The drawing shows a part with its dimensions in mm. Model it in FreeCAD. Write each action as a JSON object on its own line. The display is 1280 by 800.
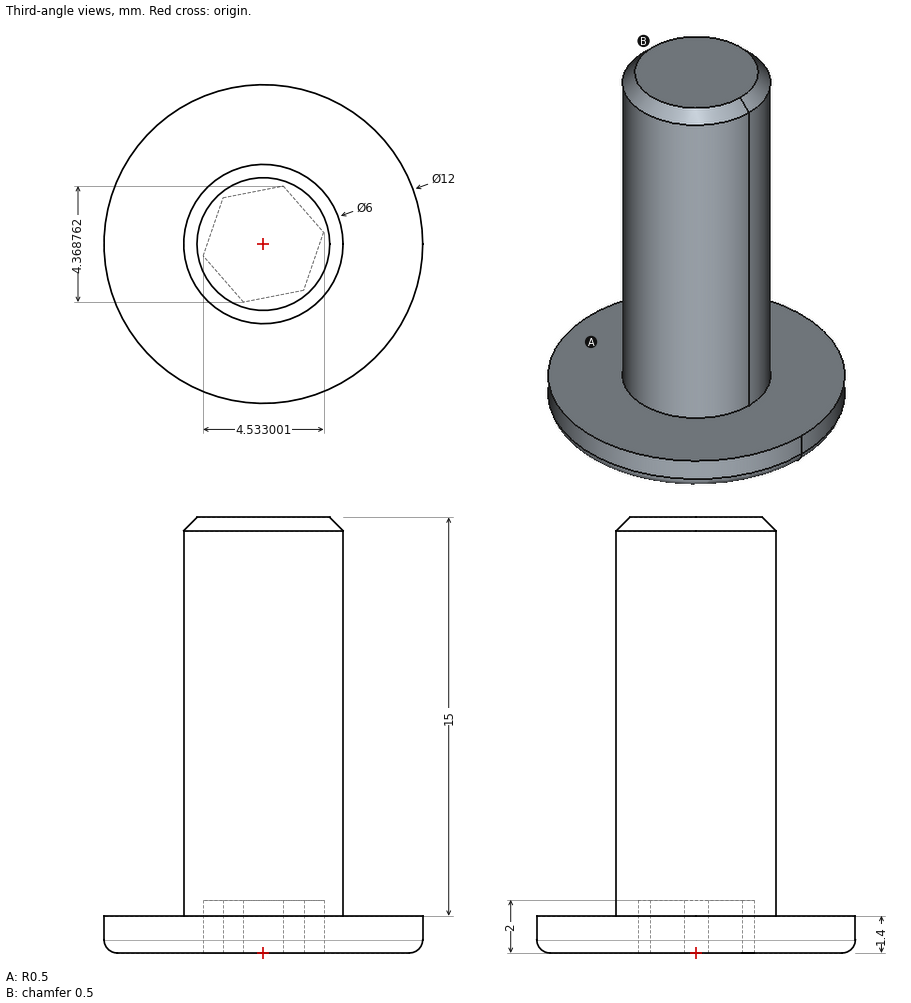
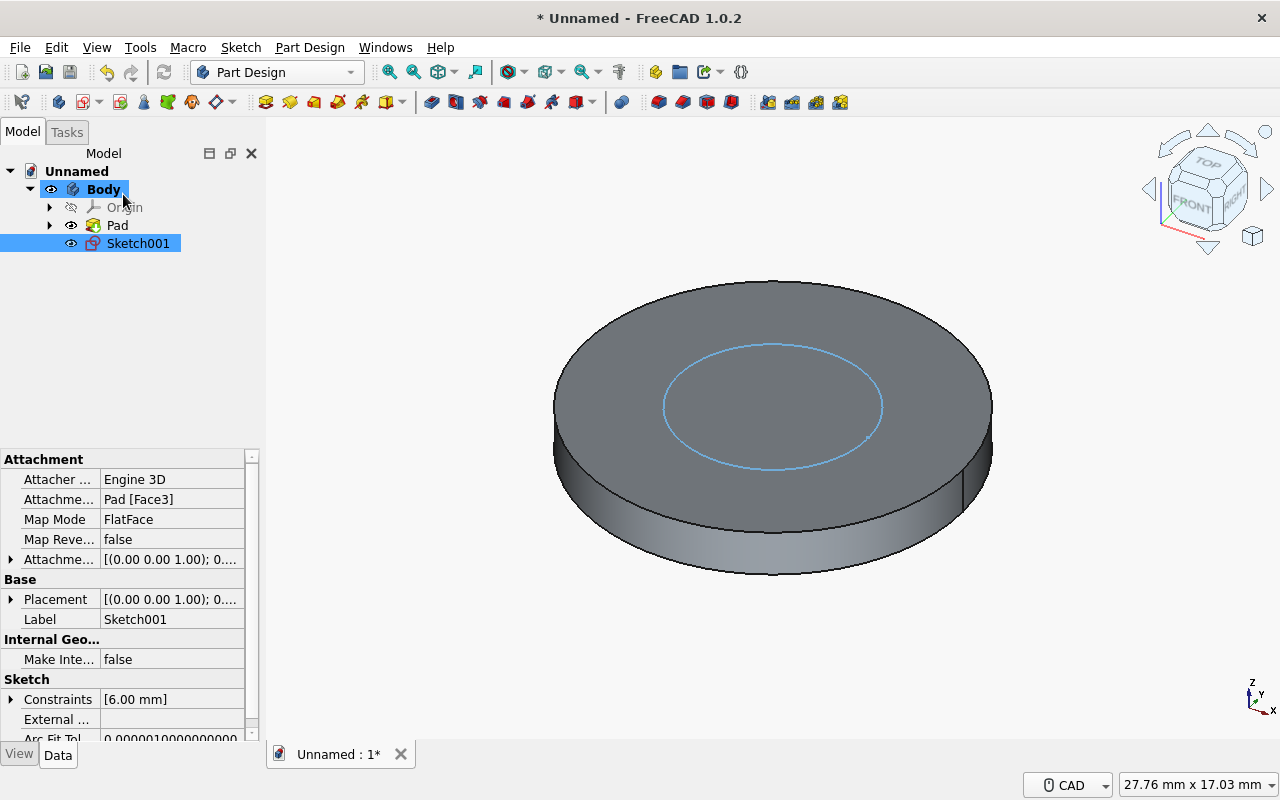
{"action": "left_click", "coordinate": [266, 102]}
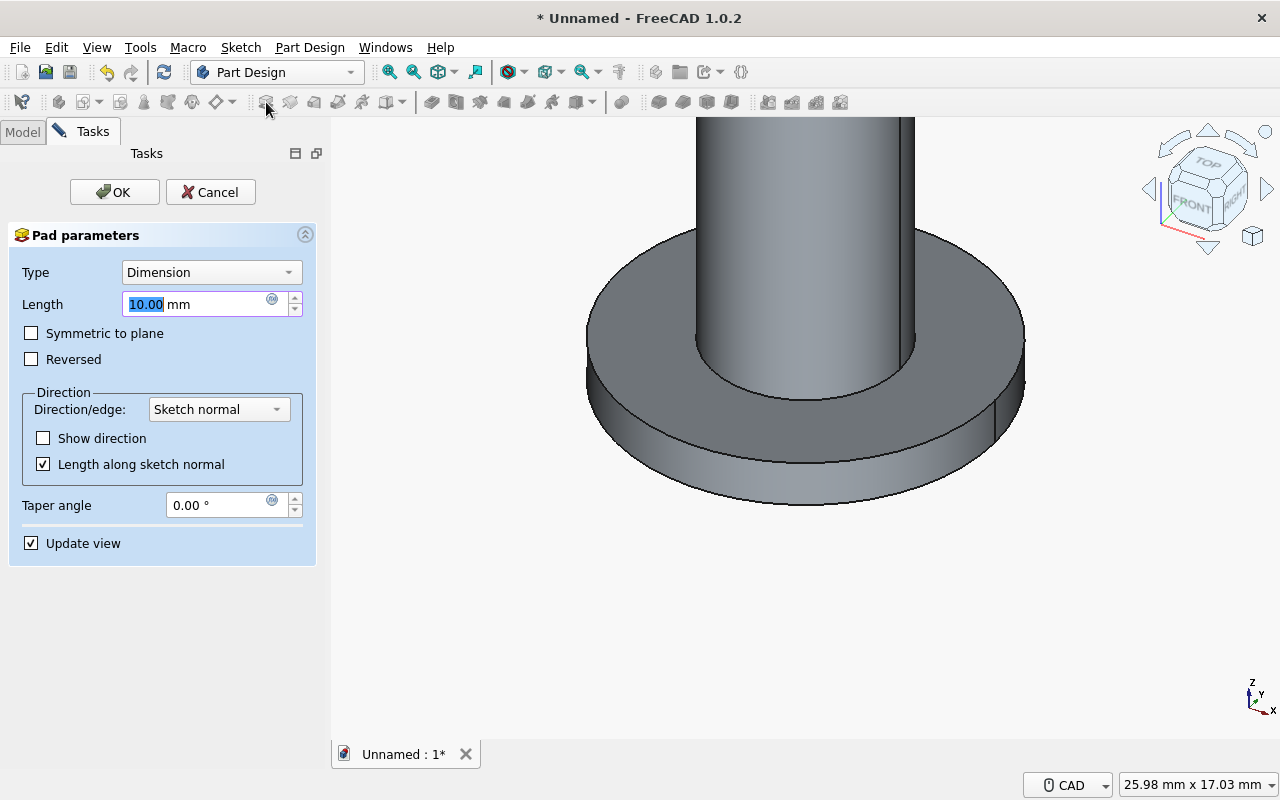
{"action": "type", "text": "15"}
{"action": "key", "text": "Tab"}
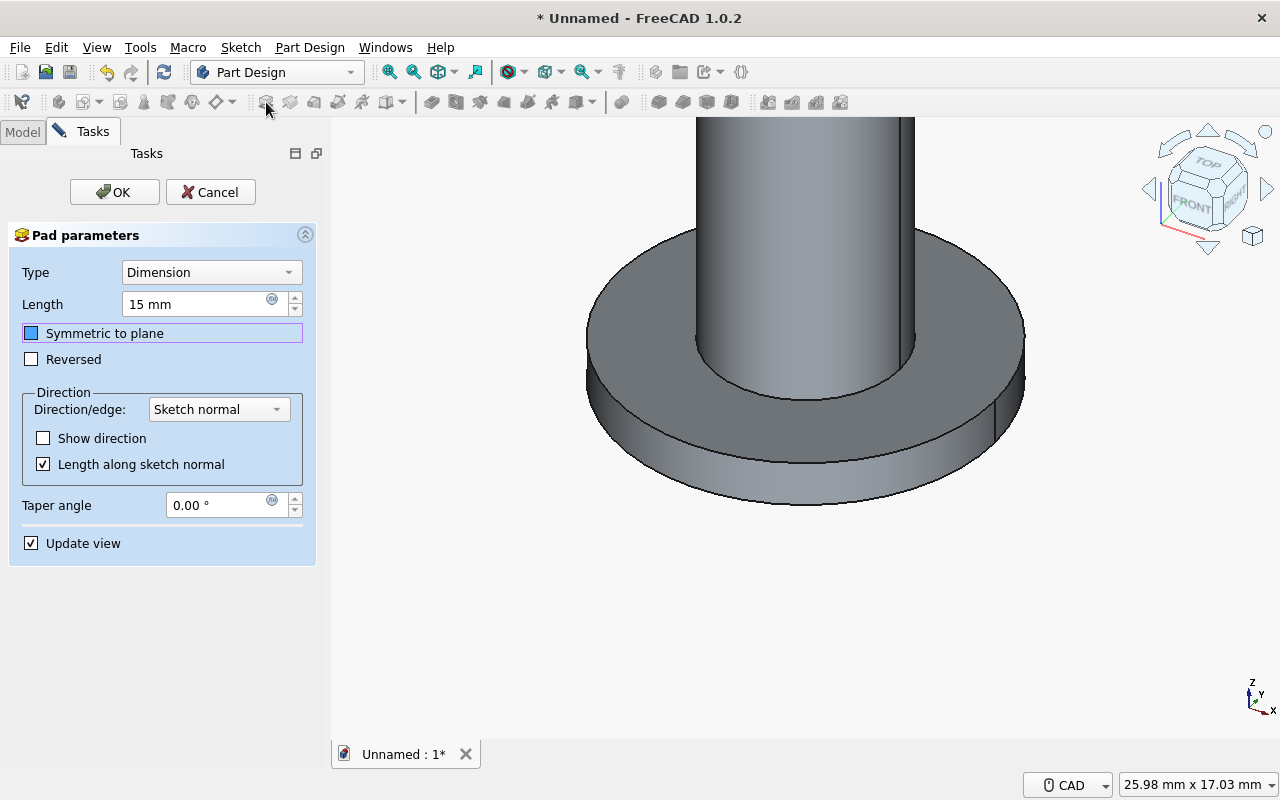
{"action": "left_click", "coordinate": [115, 192]}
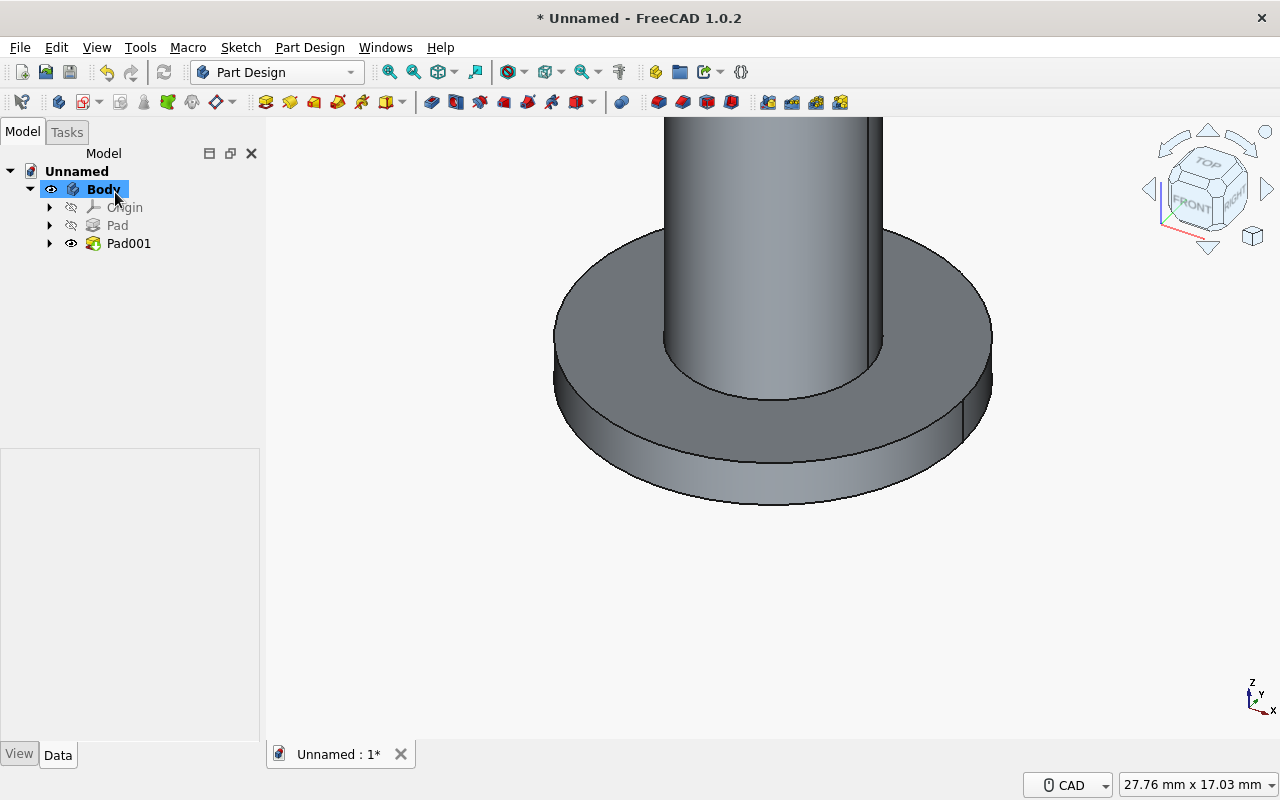
{"action": "left_click", "coordinate": [390, 72]}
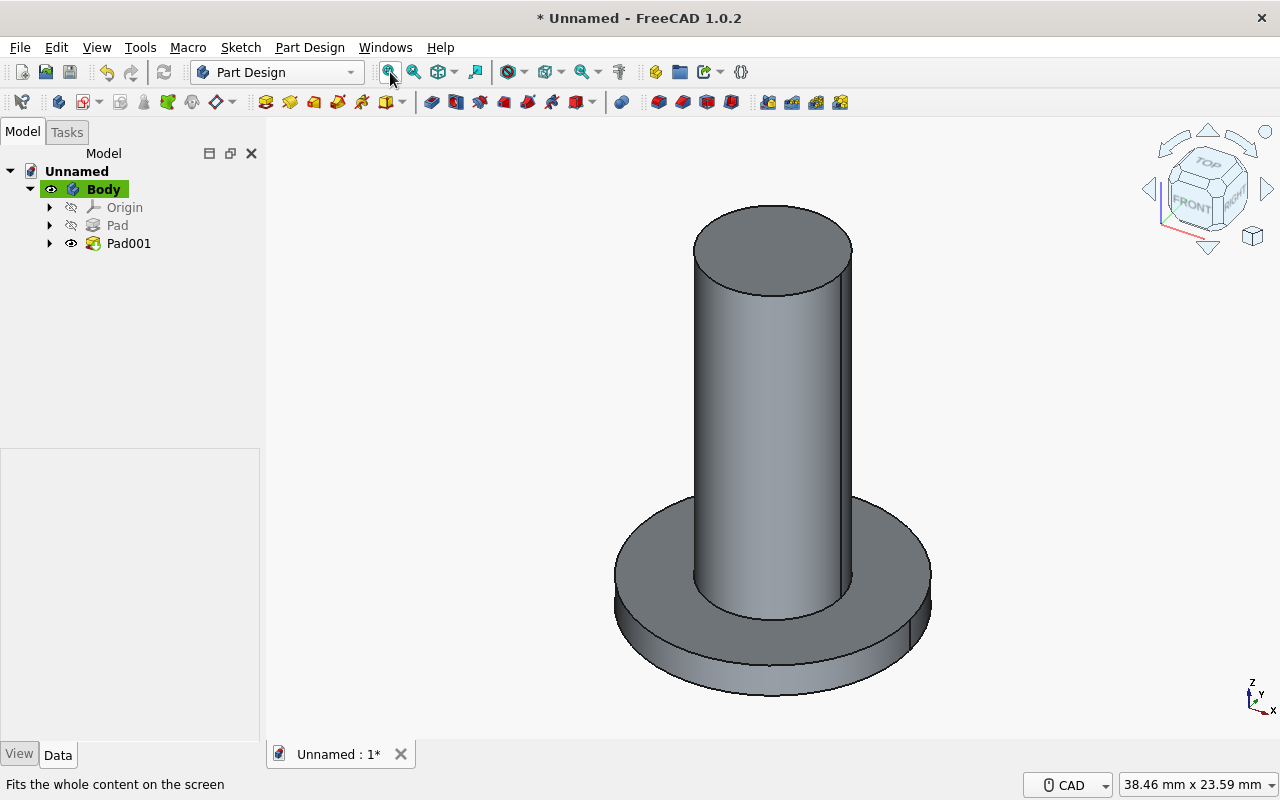
{"action": "key", "text": "0"}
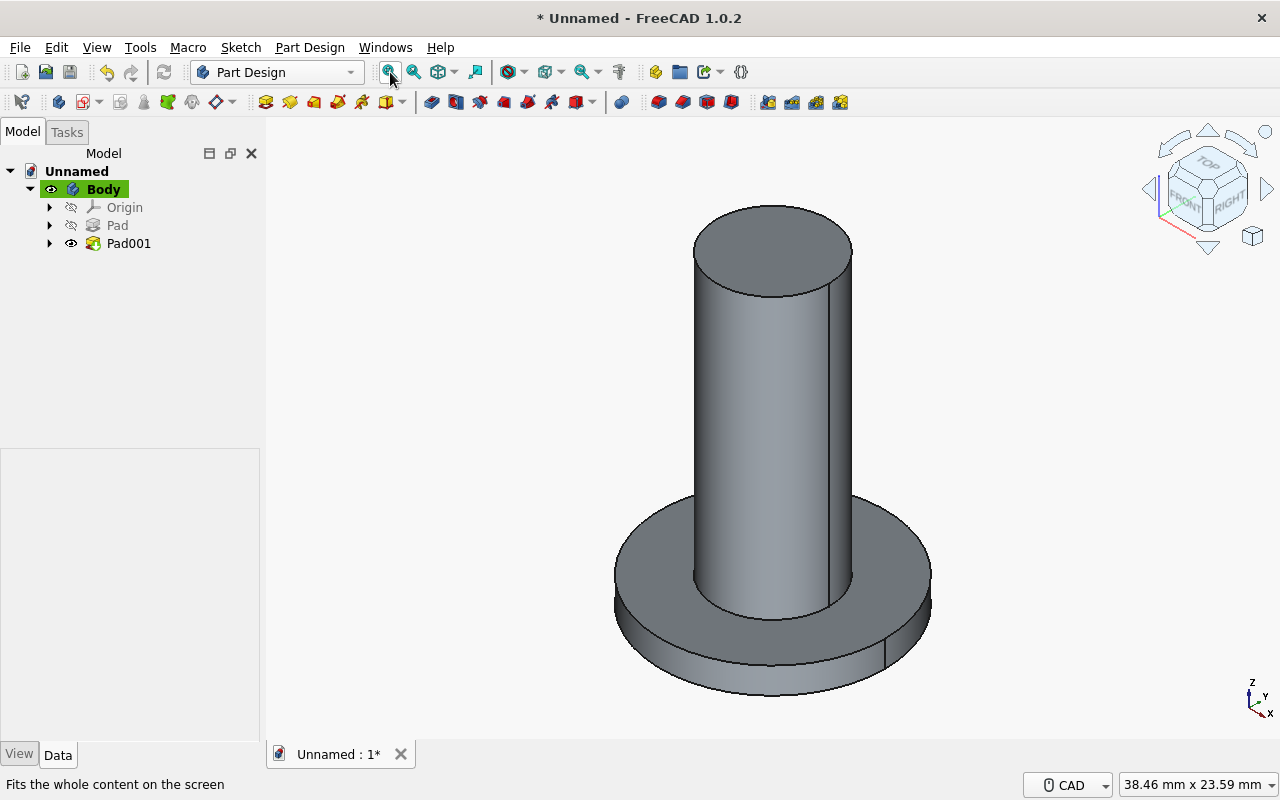
{"action": "key", "text": "2"}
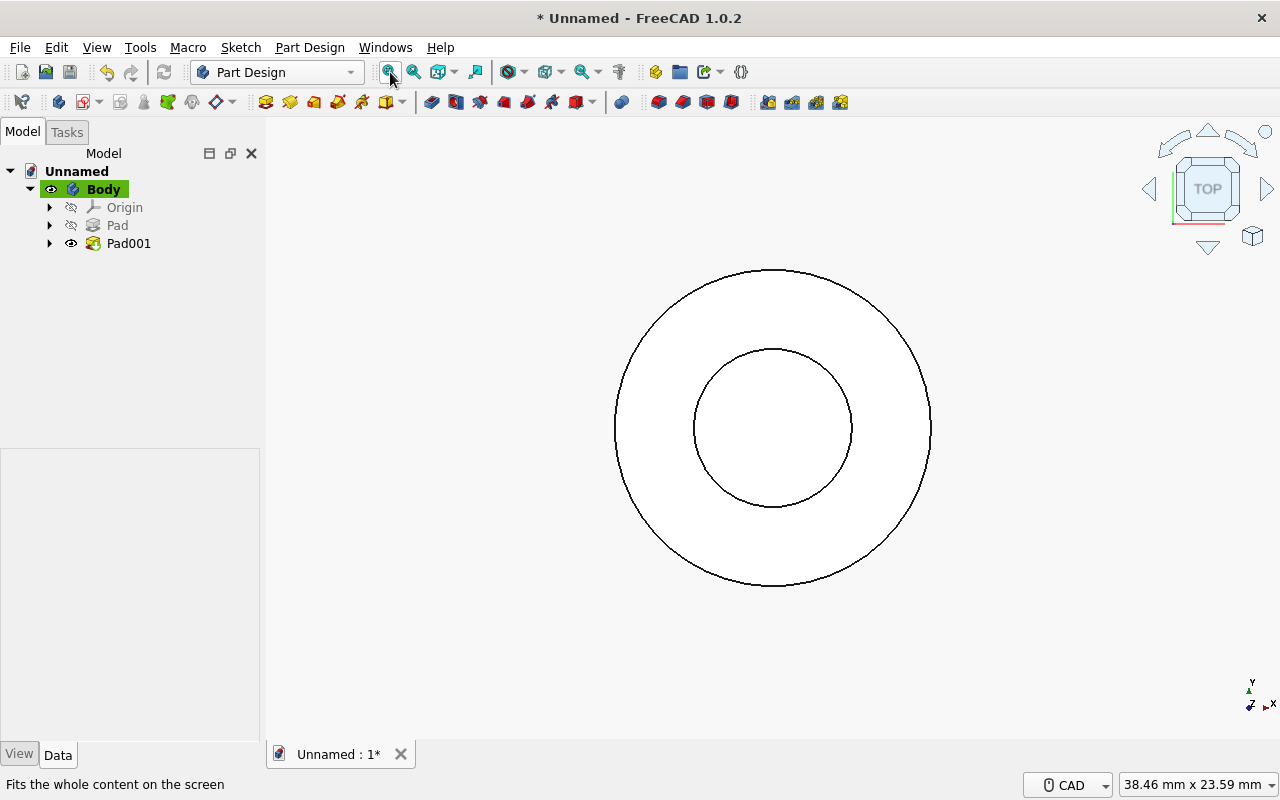
{"action": "key", "text": "1"}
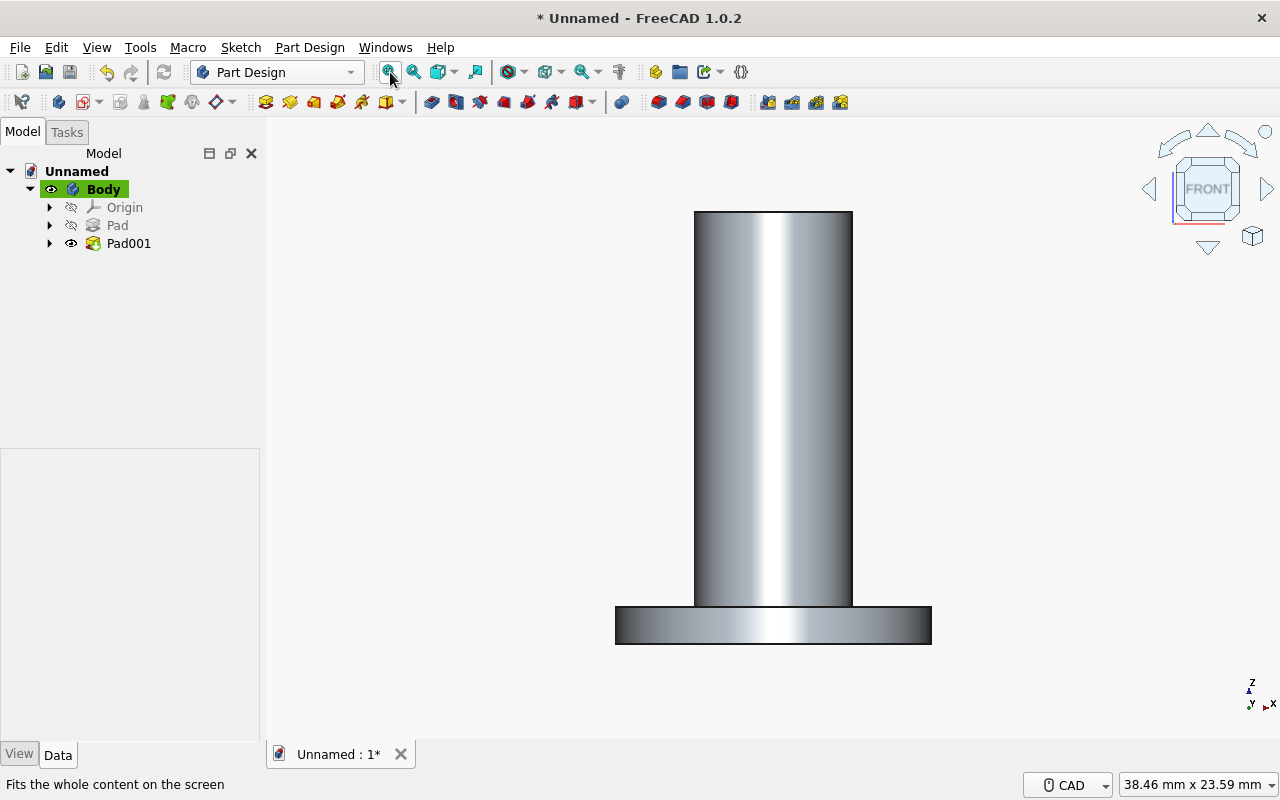
{"action": "left_click", "coordinate": [645, 643]}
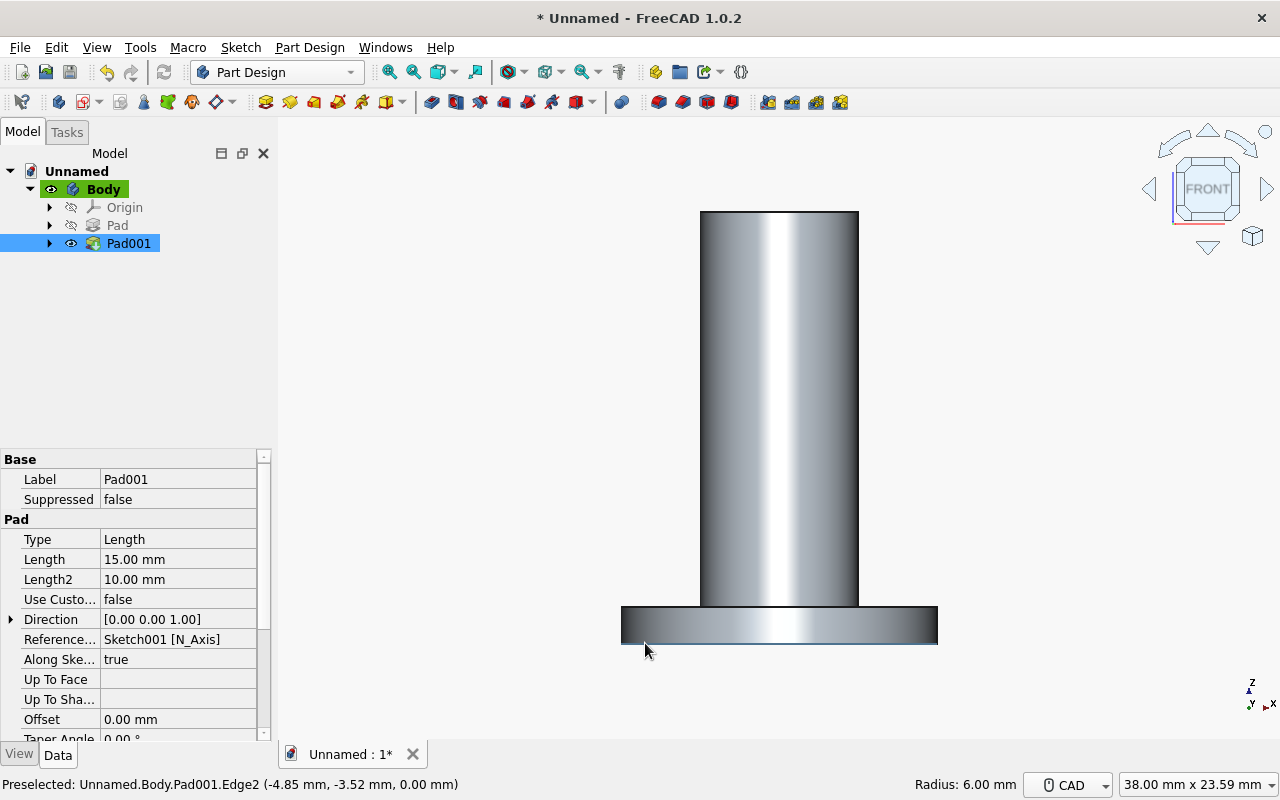
{"action": "left_click", "coordinate": [660, 102]}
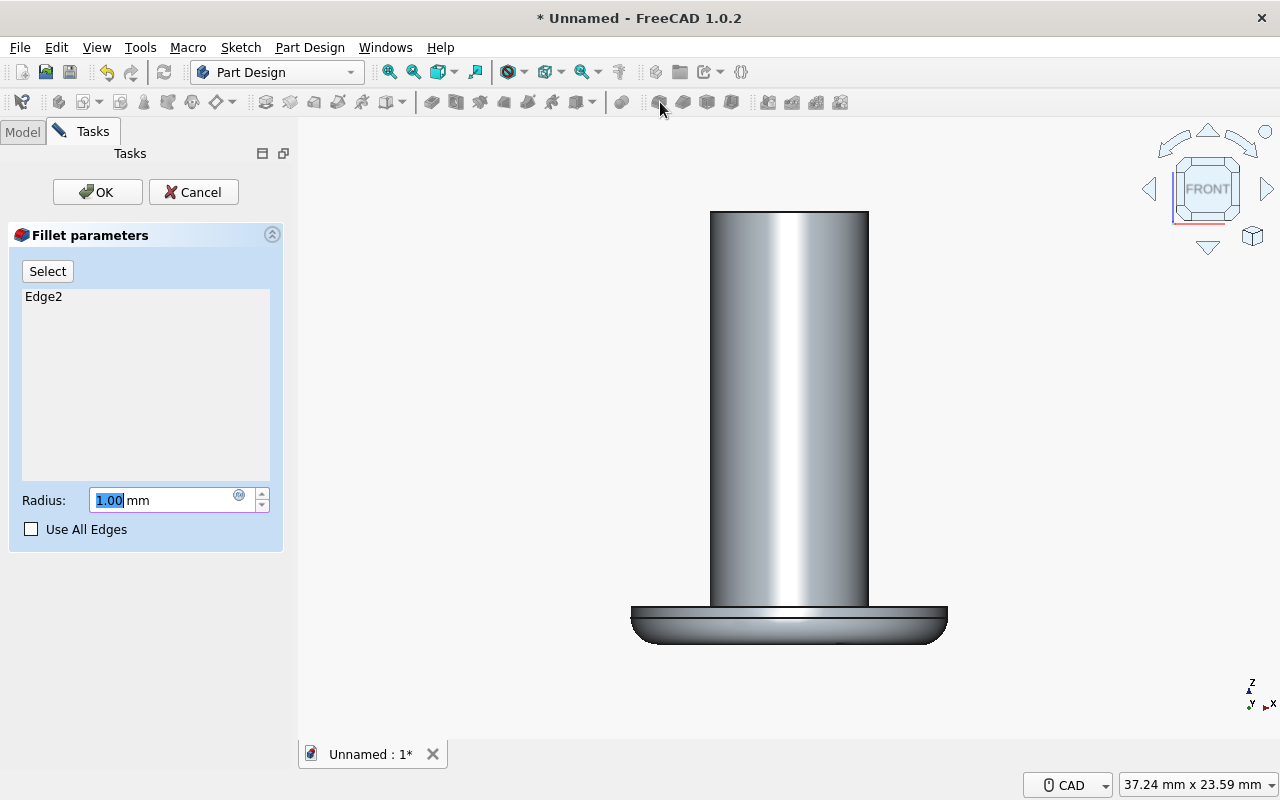
{"action": "type", "text": "0.5"}
{"action": "key", "text": "Tab"}